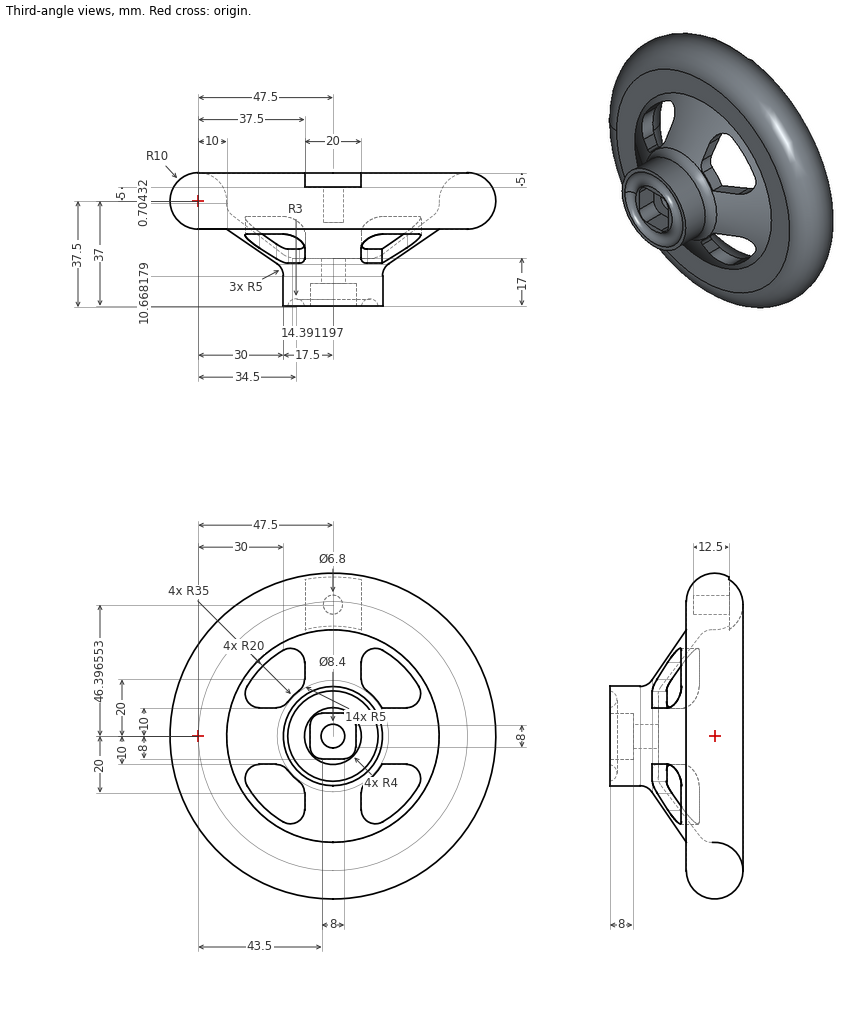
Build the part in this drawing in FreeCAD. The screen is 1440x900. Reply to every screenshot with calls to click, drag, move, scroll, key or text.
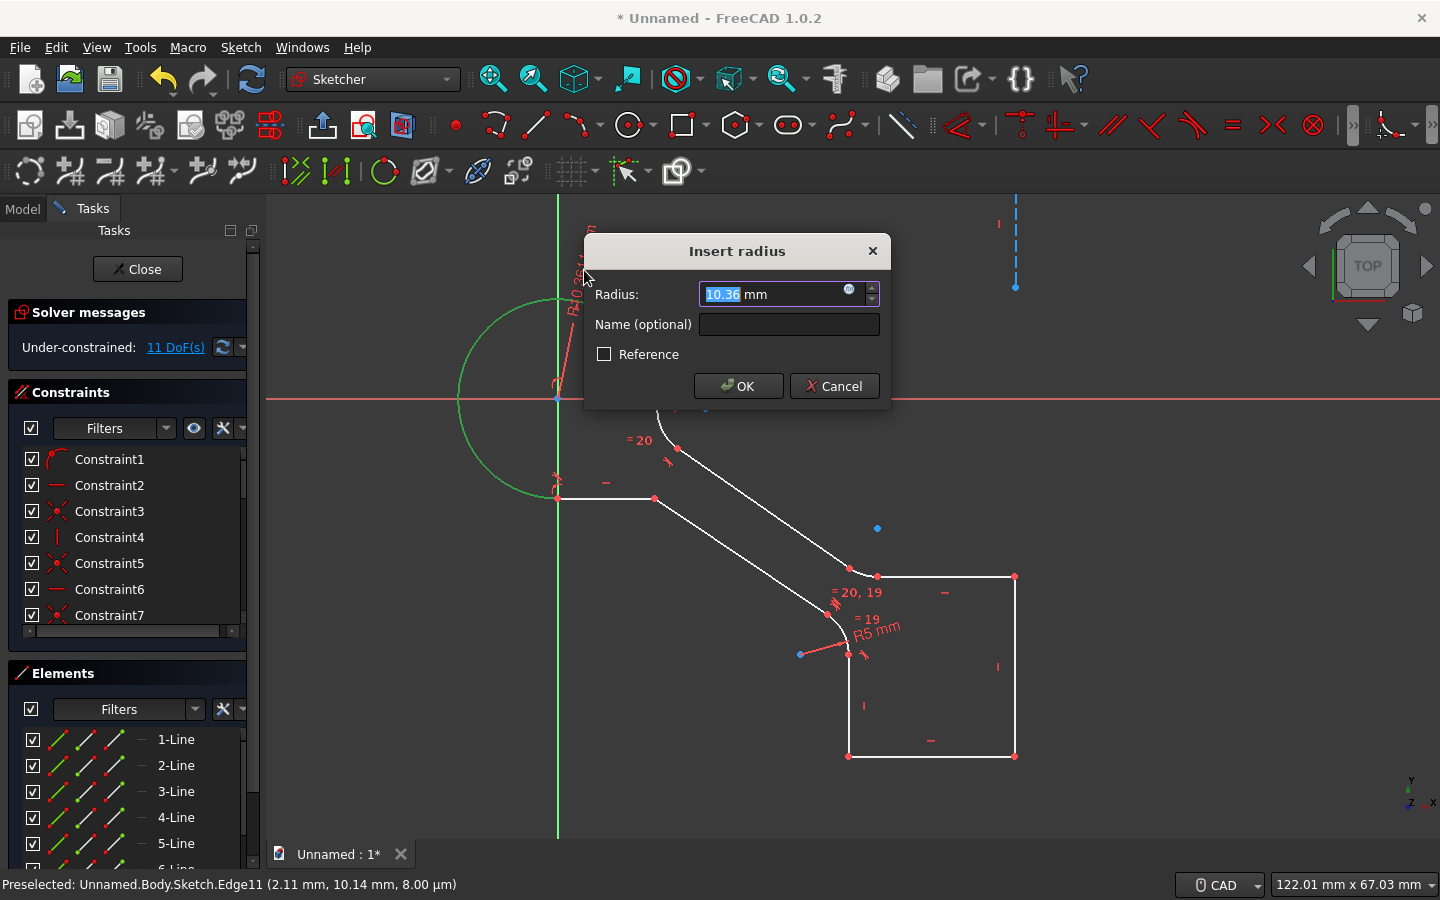
text(10)
key(Return)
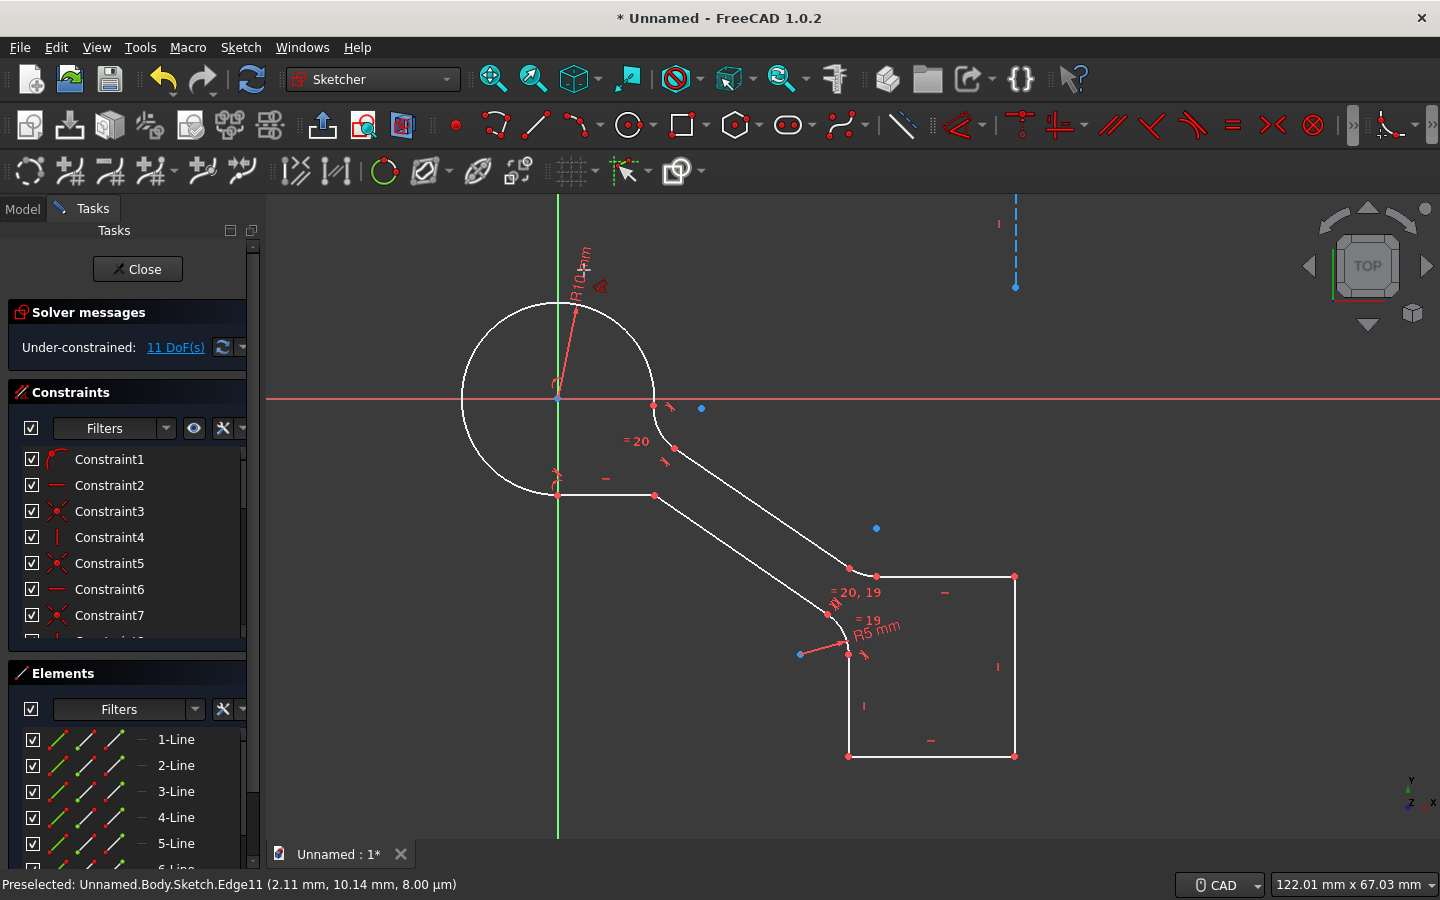
click(587, 495)
click(606, 529)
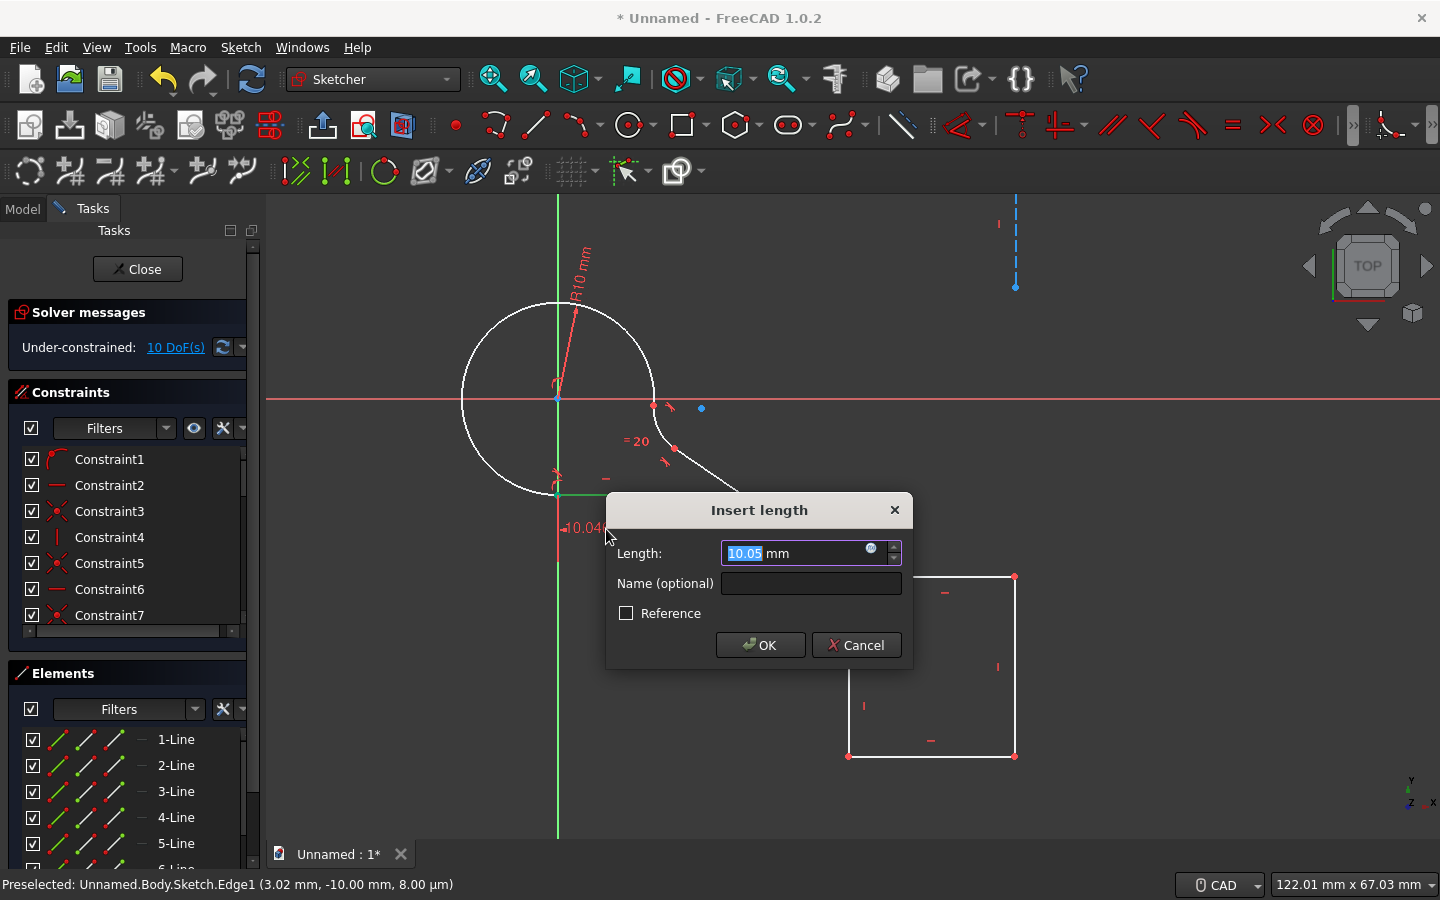
text(10)
key(Return)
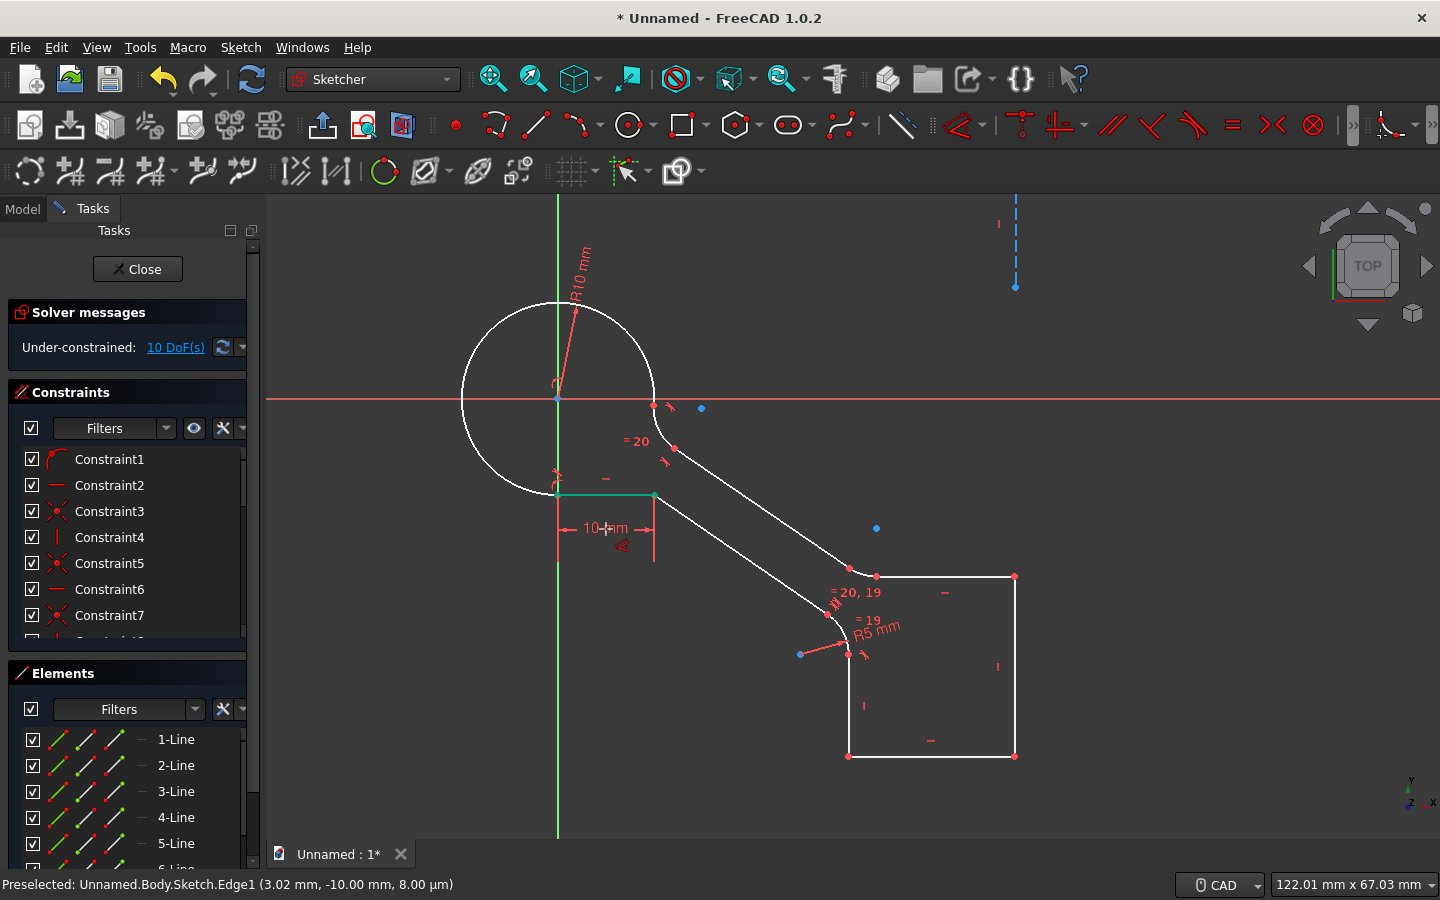
click(1015, 703)
click(1049, 667)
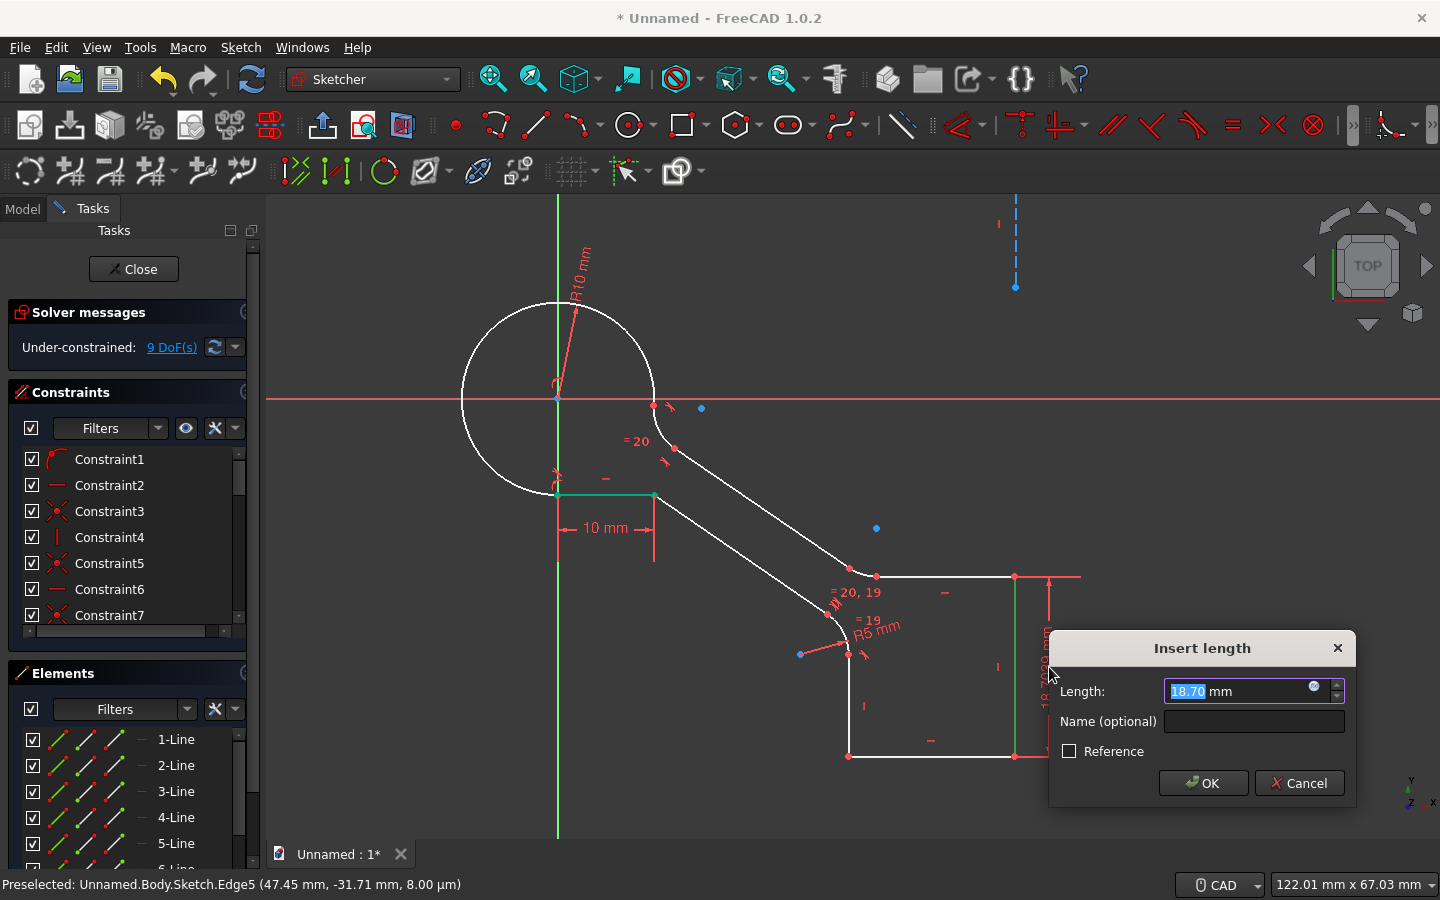
text(17)
key(Return)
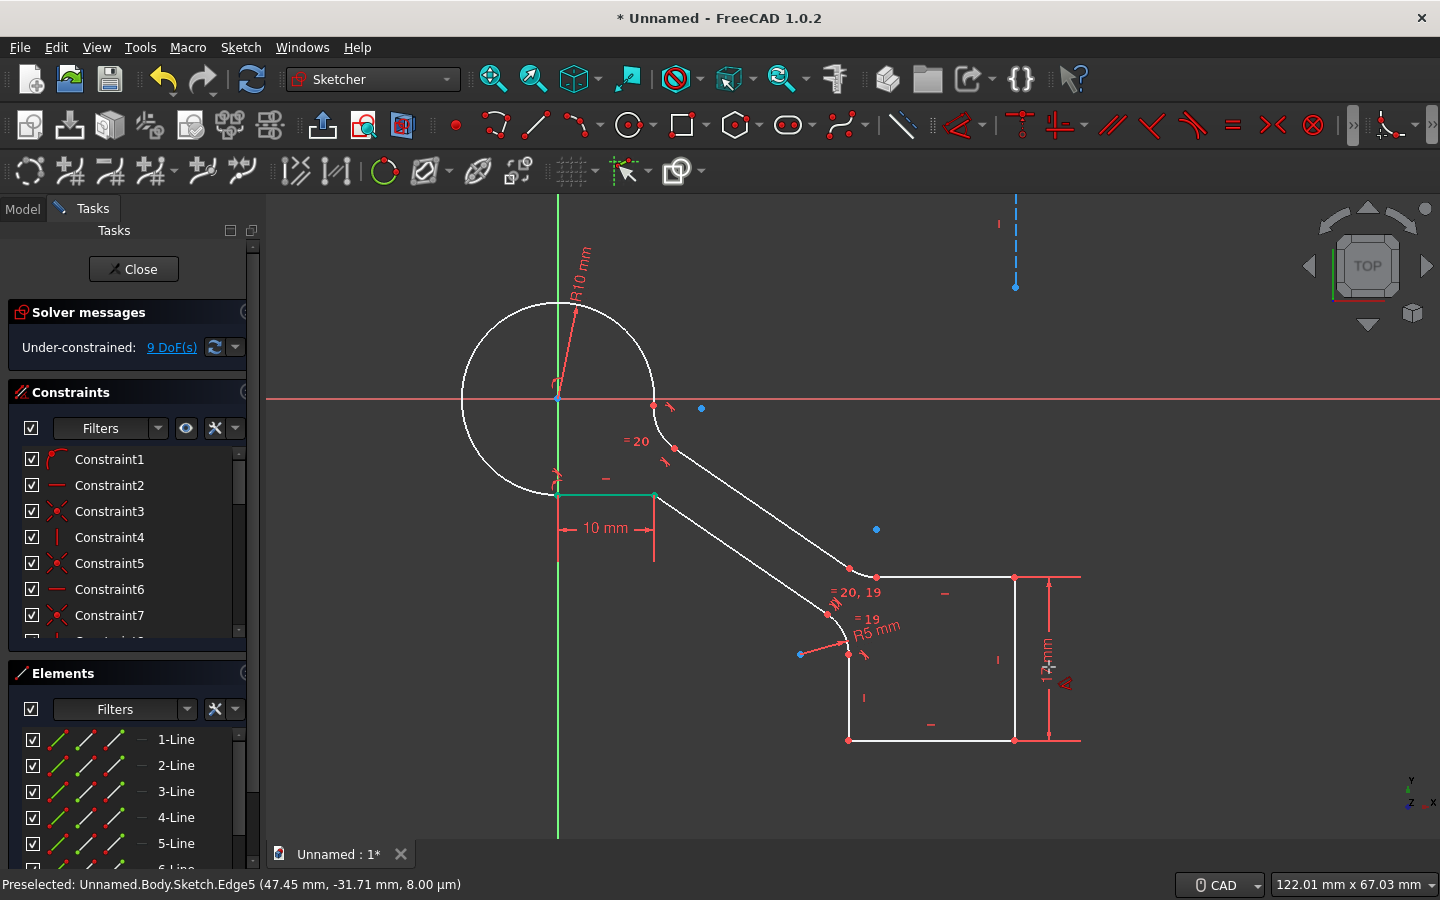
click(849, 654)
click(703, 688)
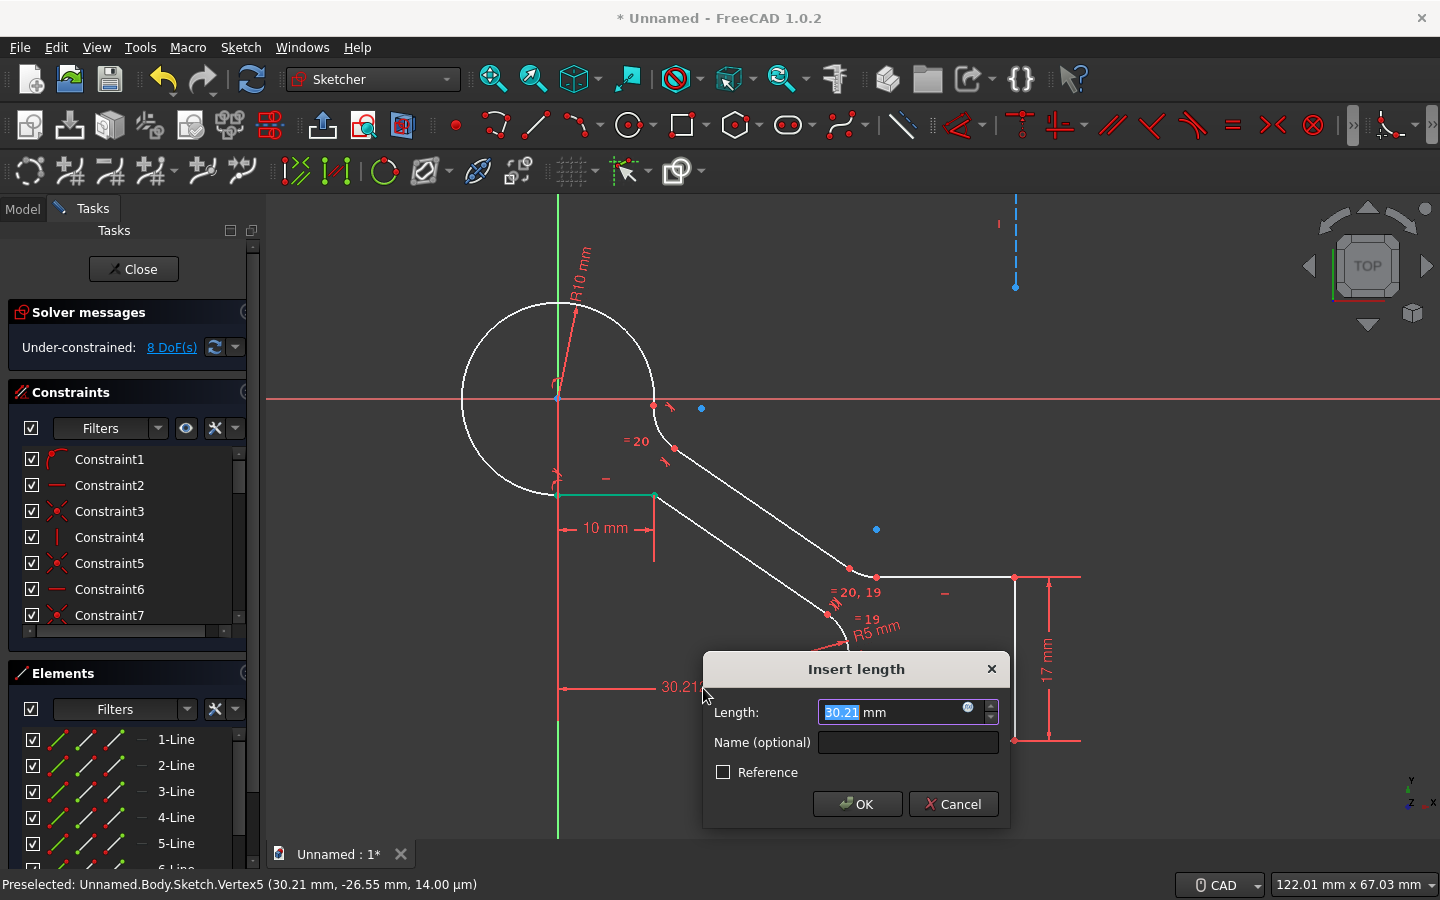
text(30)
key(Return)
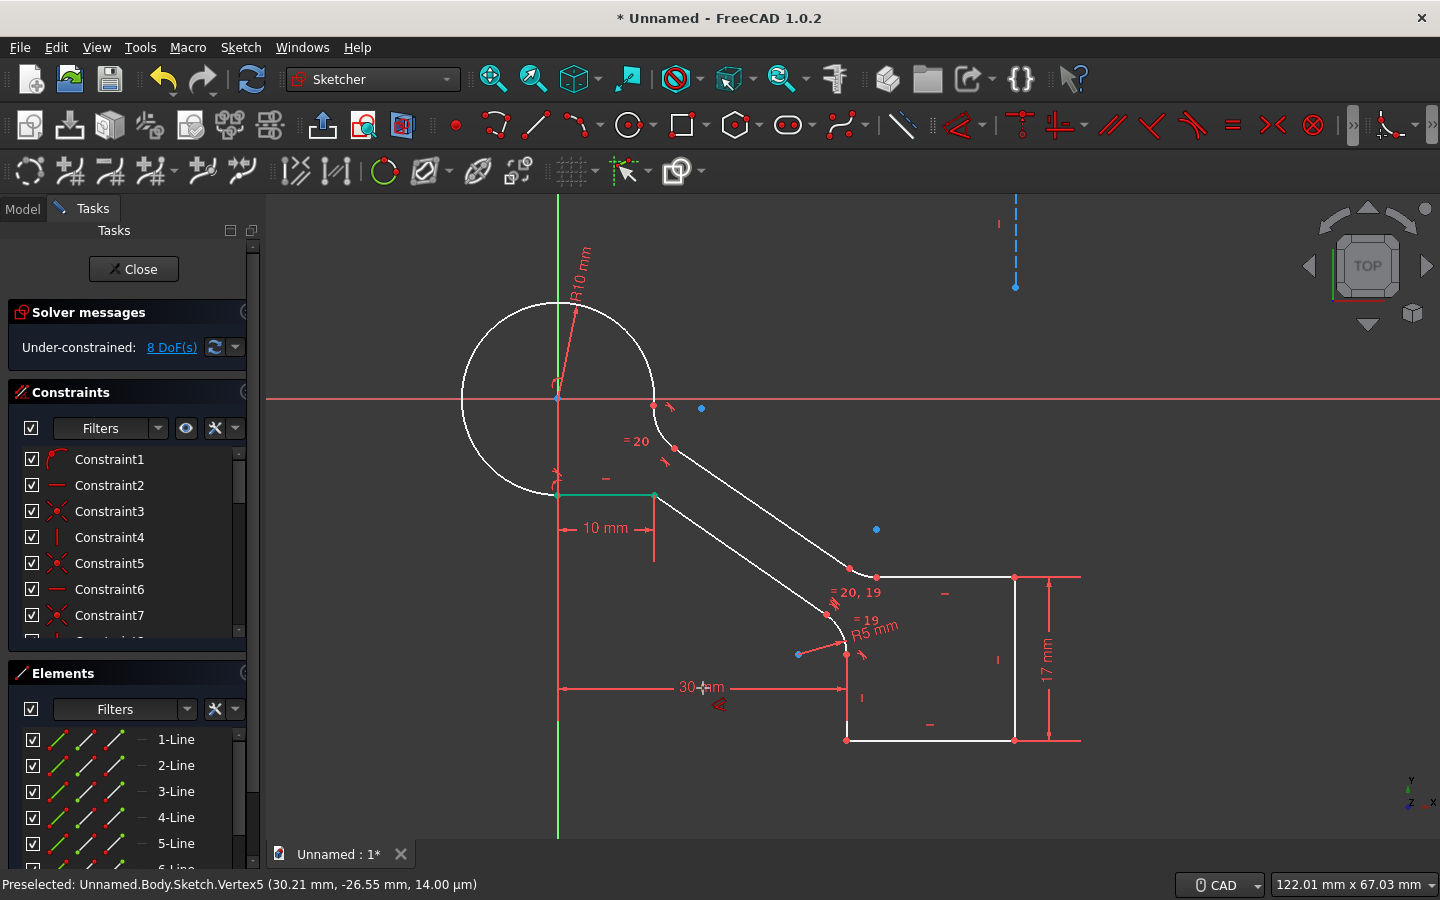
click(847, 741)
click(524, 570)